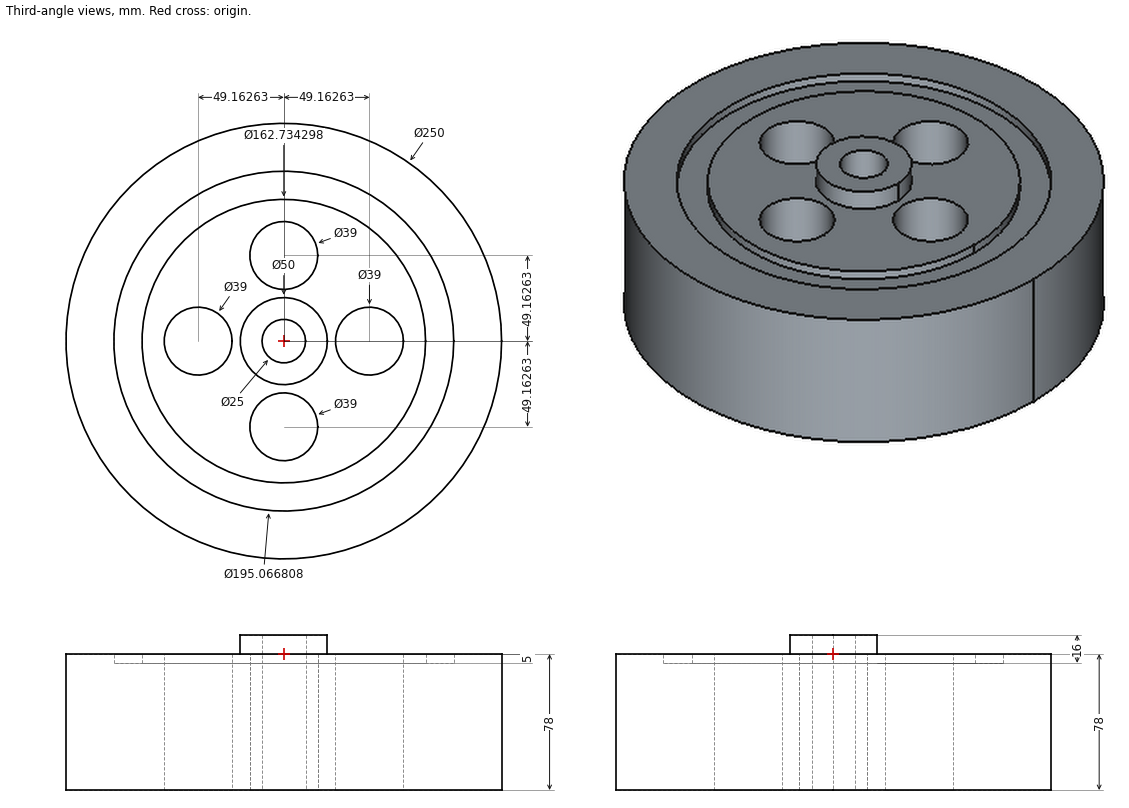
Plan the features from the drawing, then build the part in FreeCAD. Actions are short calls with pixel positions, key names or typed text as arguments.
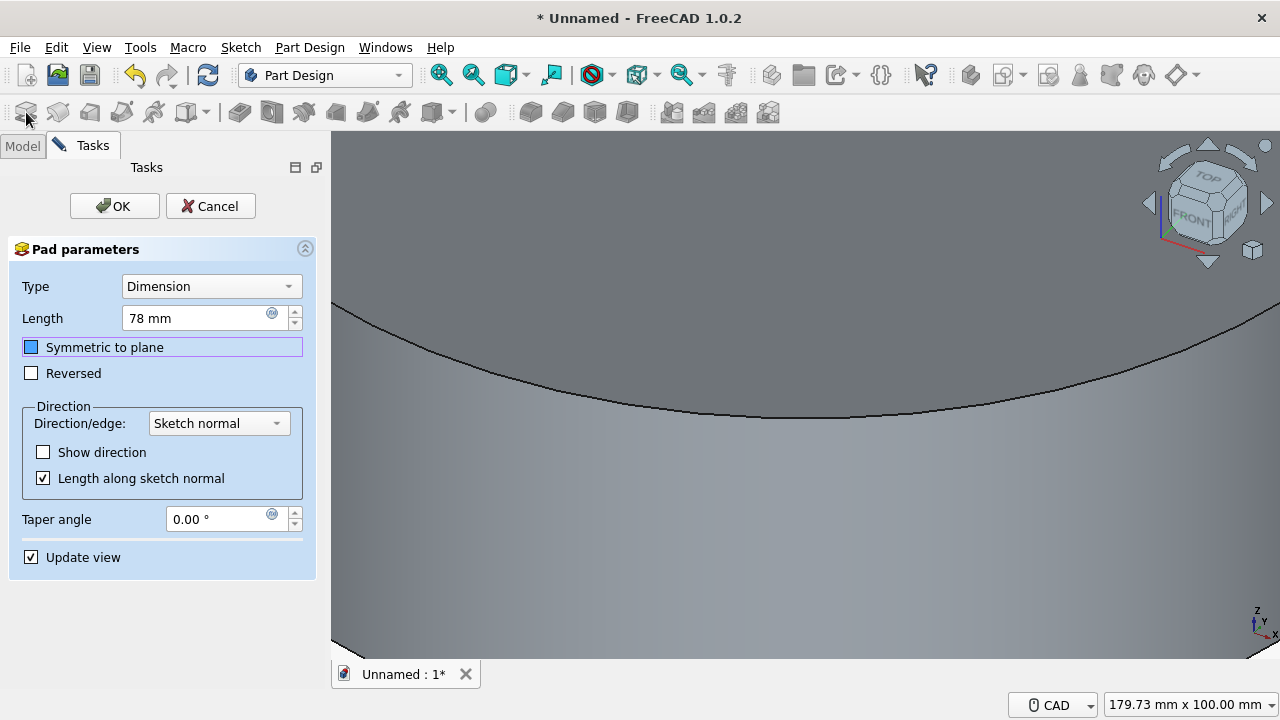
click(30, 373)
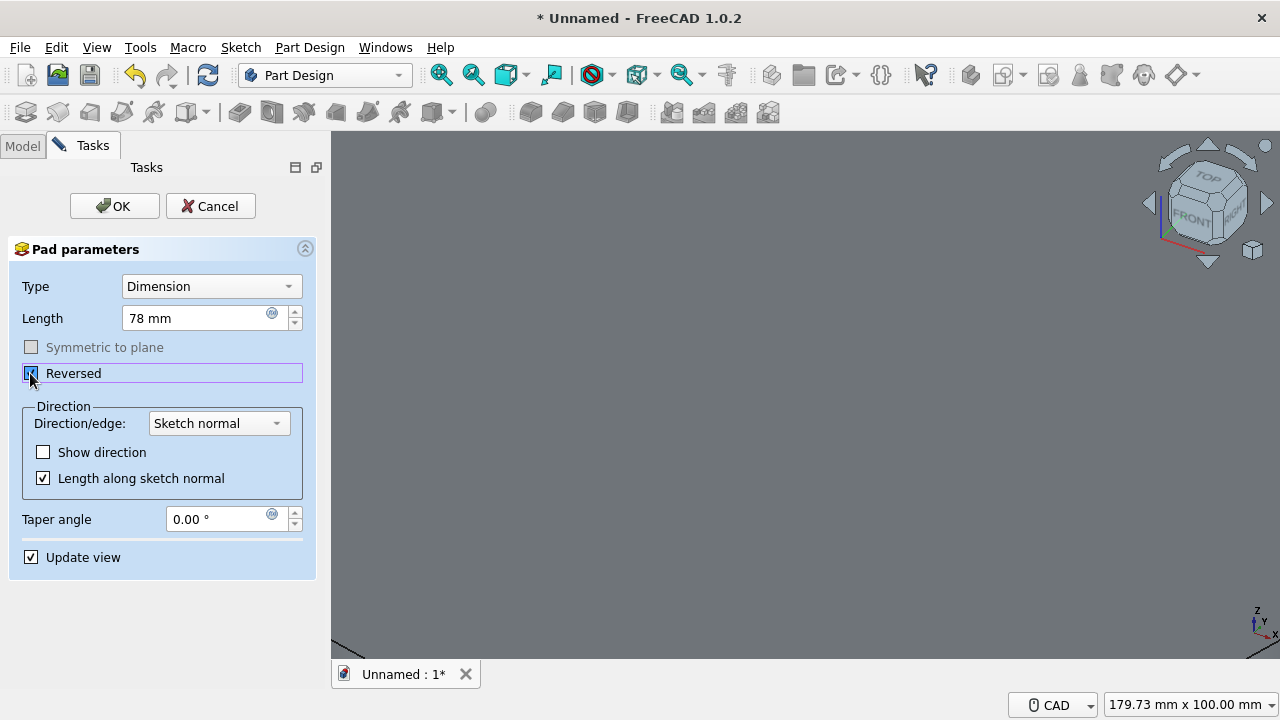
click(115, 206)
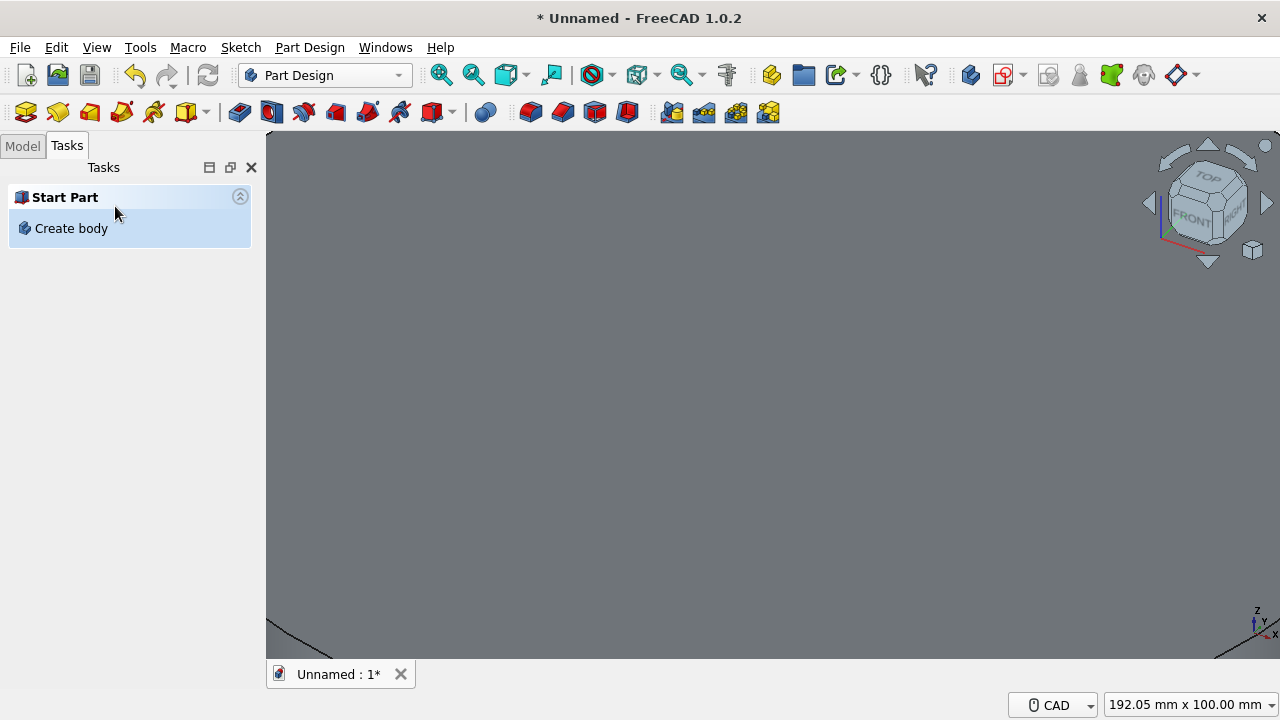
click(442, 76)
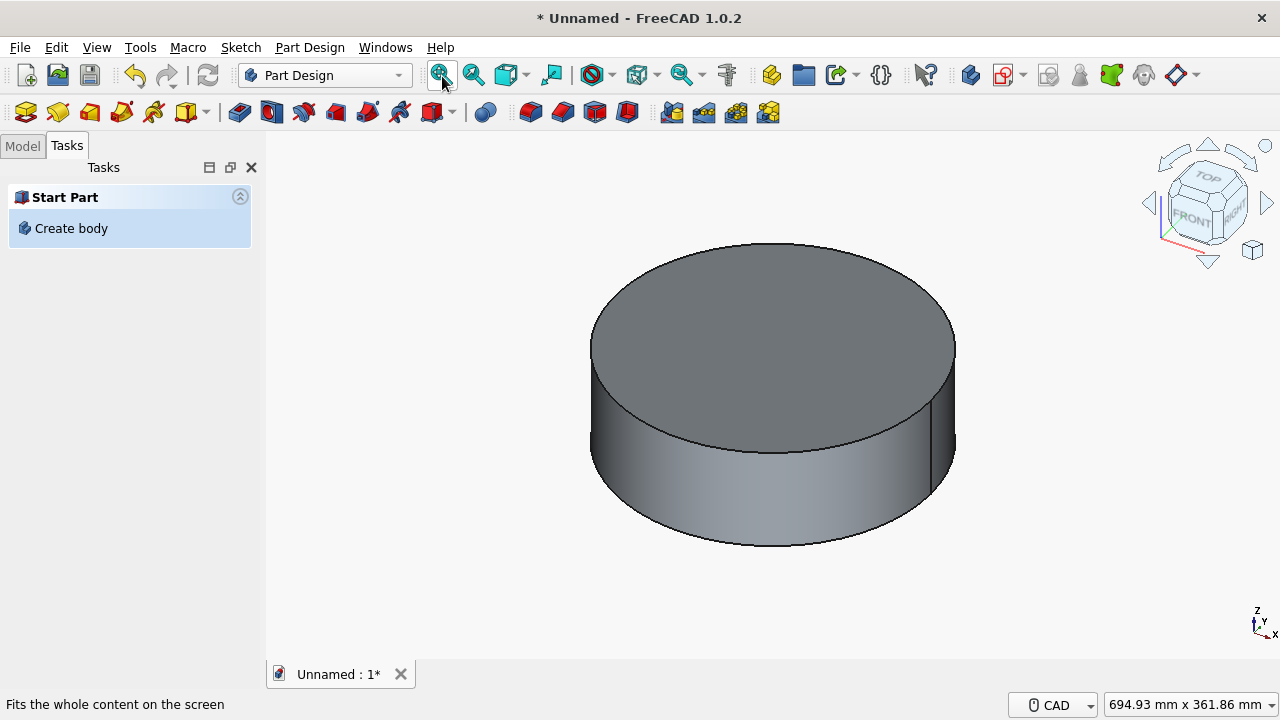
click(1004, 76)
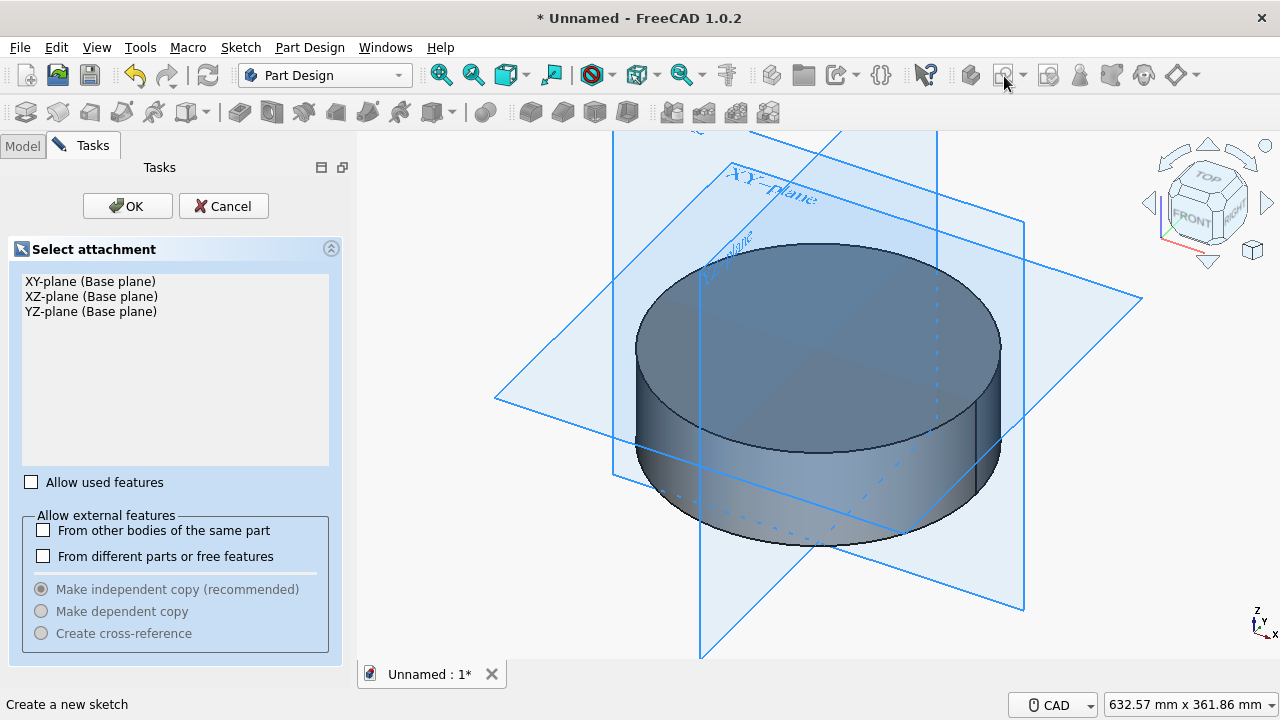
click(82, 282)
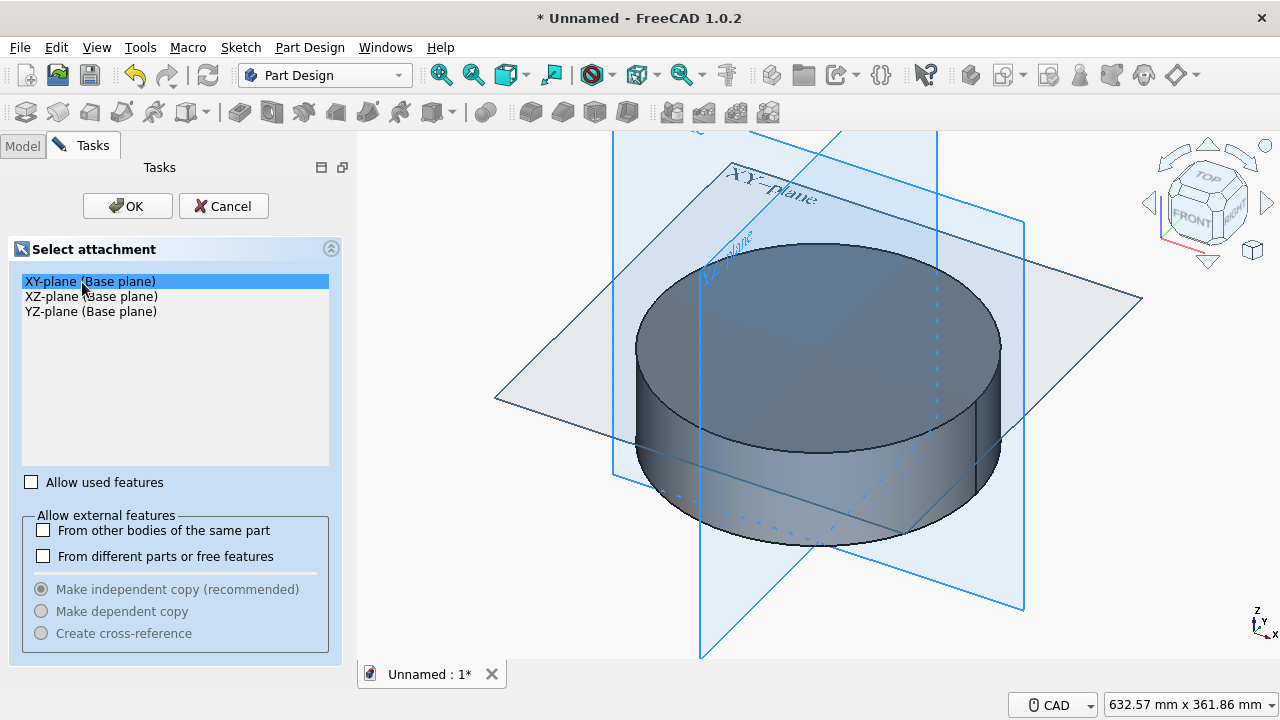
click(128, 206)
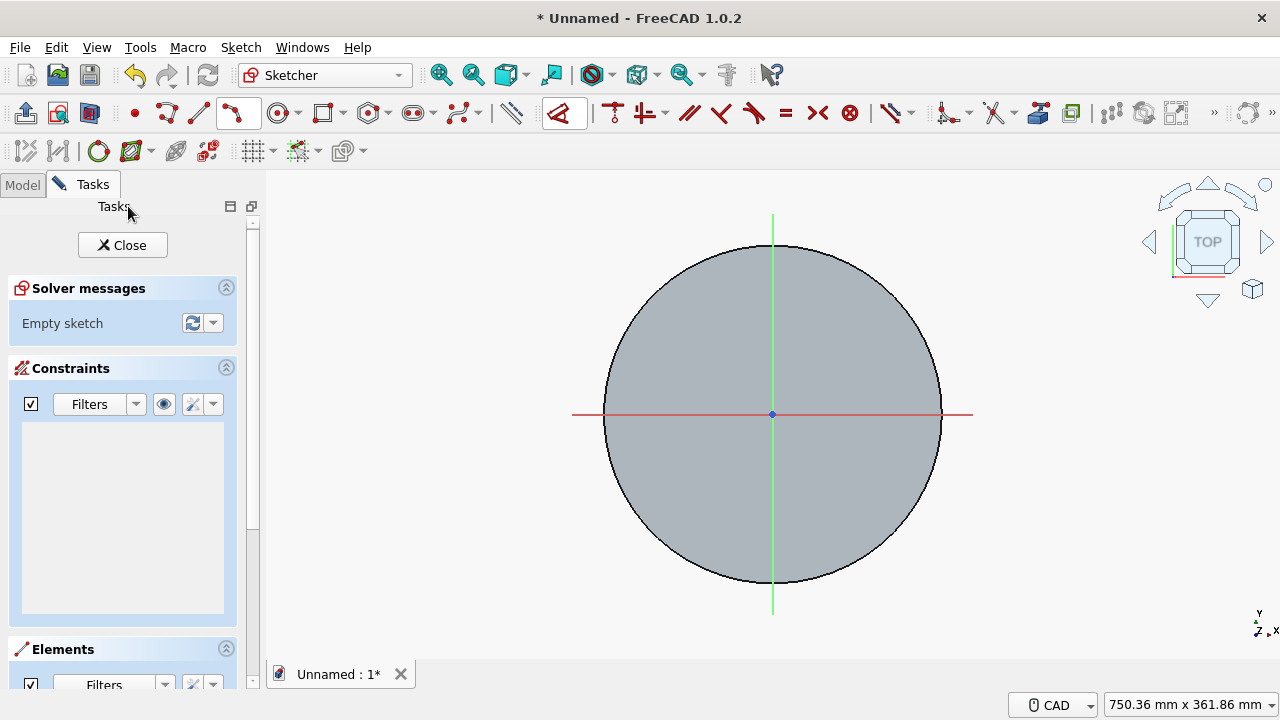
click(278, 114)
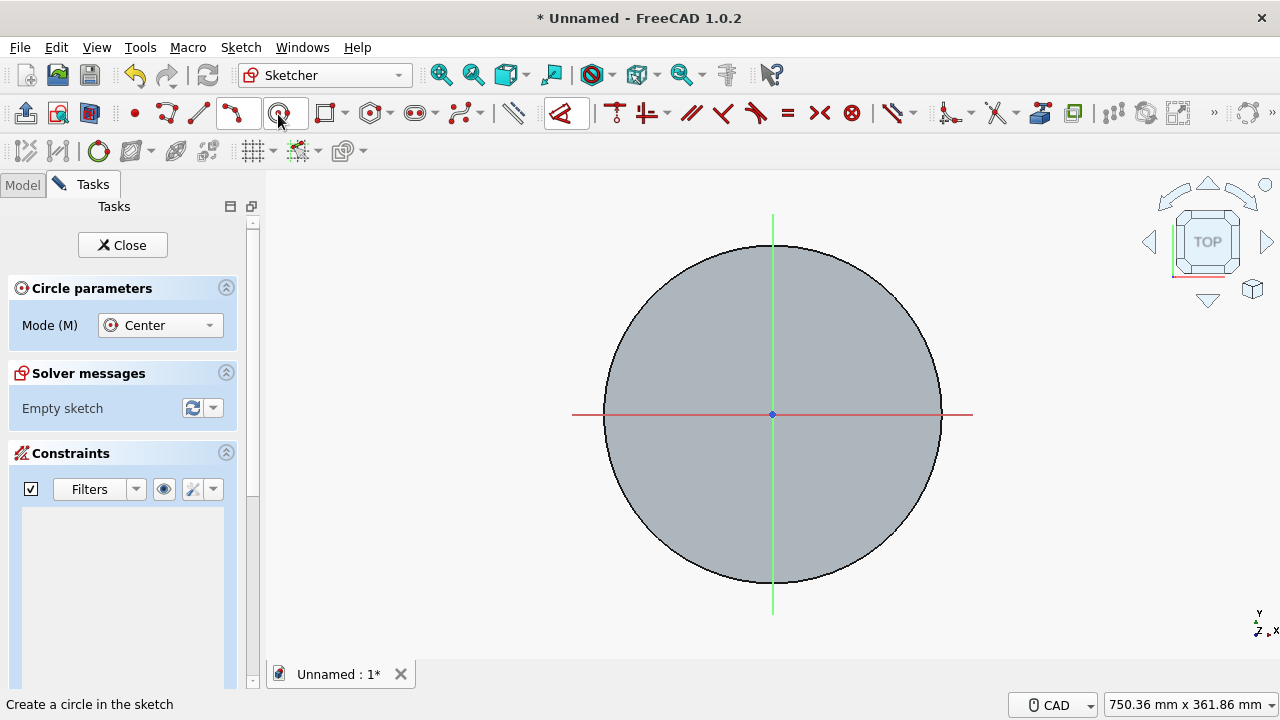
click(773, 414)
move(866, 321)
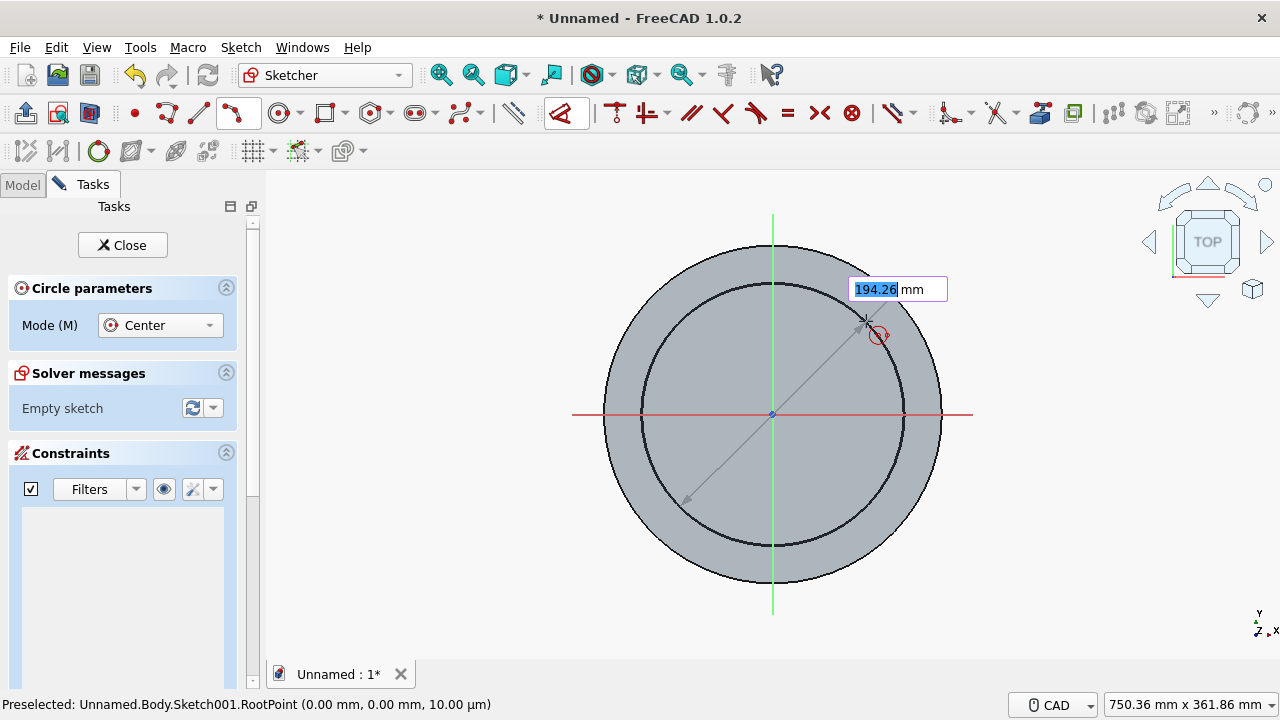
text(195.066808)
key(Return)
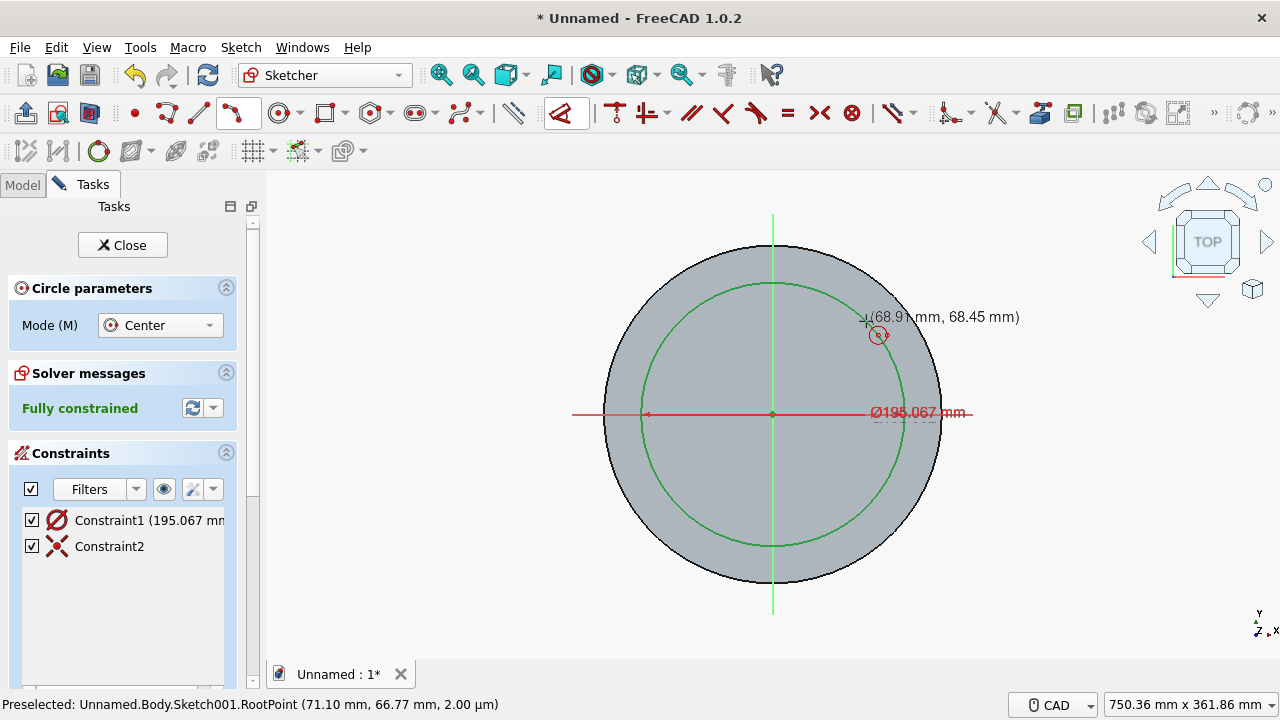
click(773, 414)
move(851, 337)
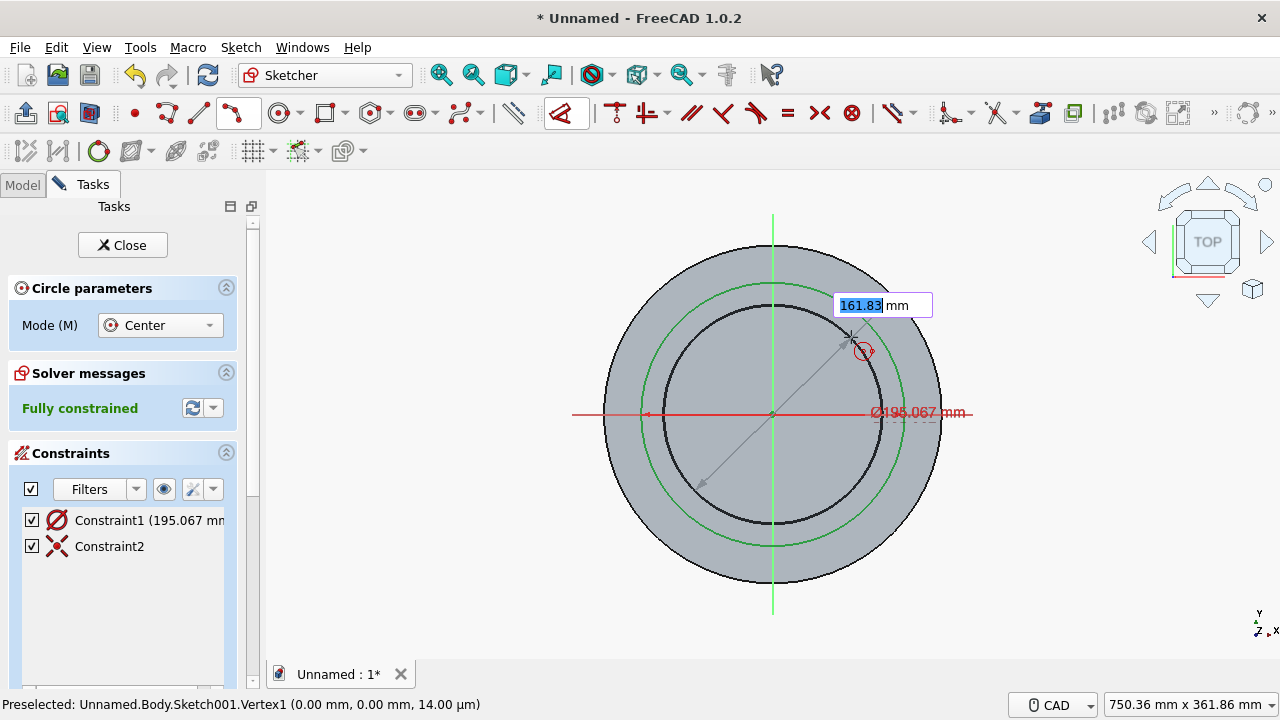
text(162.734298)
key(Return)
key(Escape)